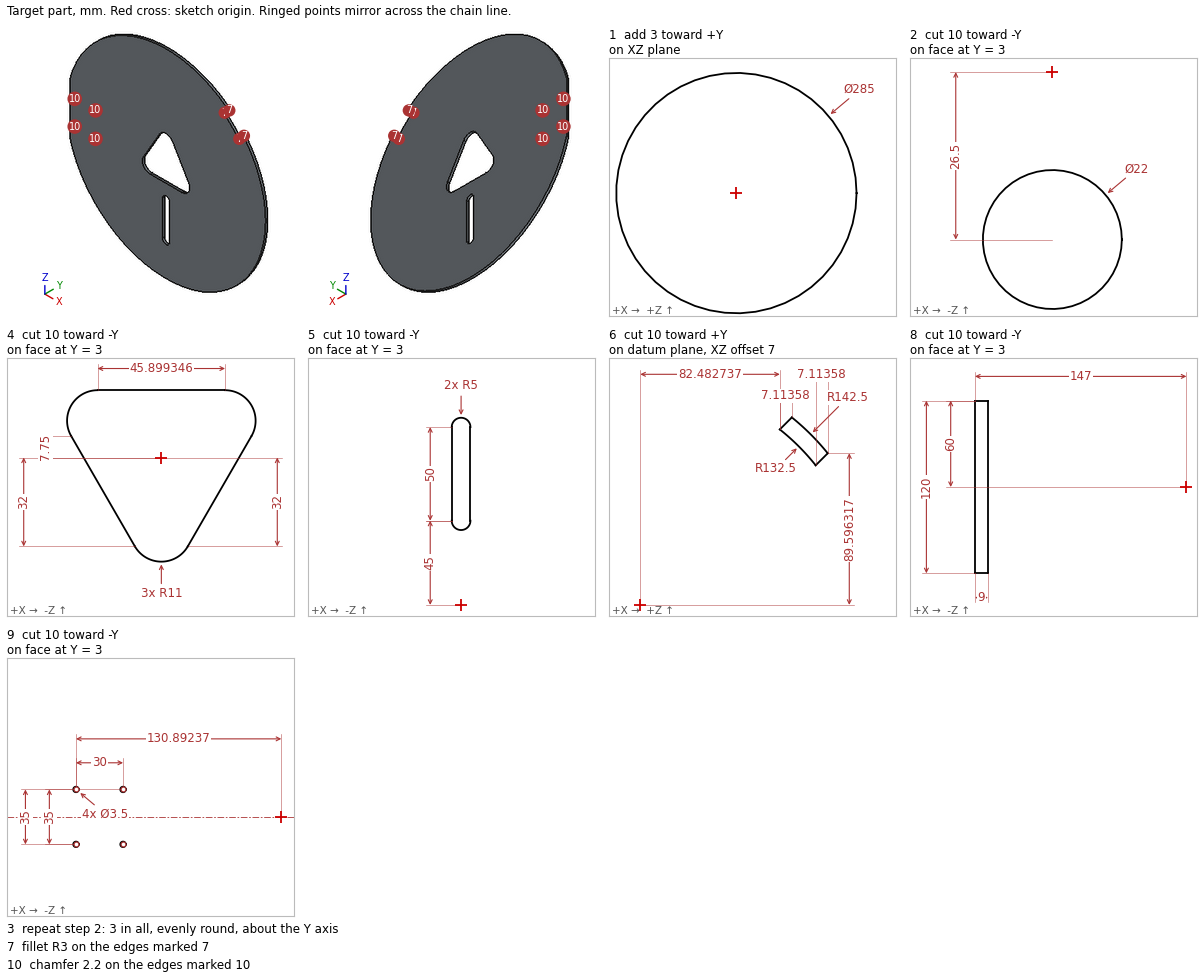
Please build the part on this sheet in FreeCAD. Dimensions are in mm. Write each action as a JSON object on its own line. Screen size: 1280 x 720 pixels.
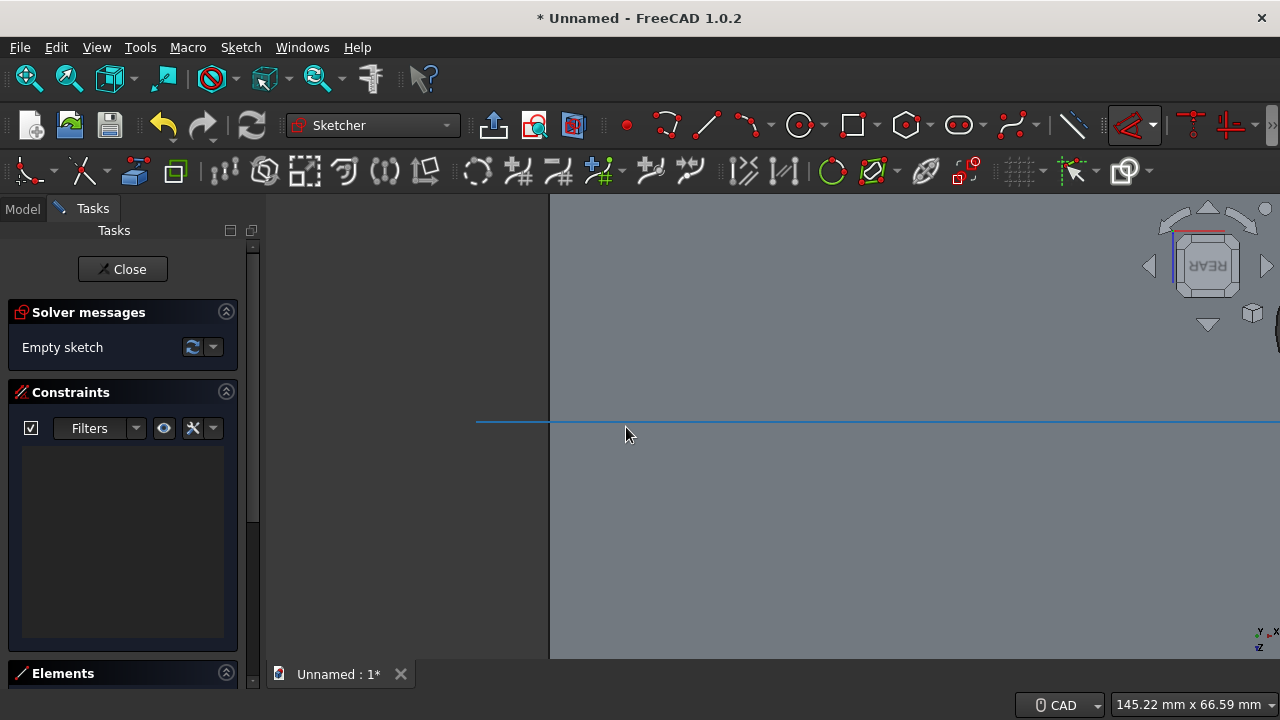
{"action": "left_click", "coordinate": [800, 126]}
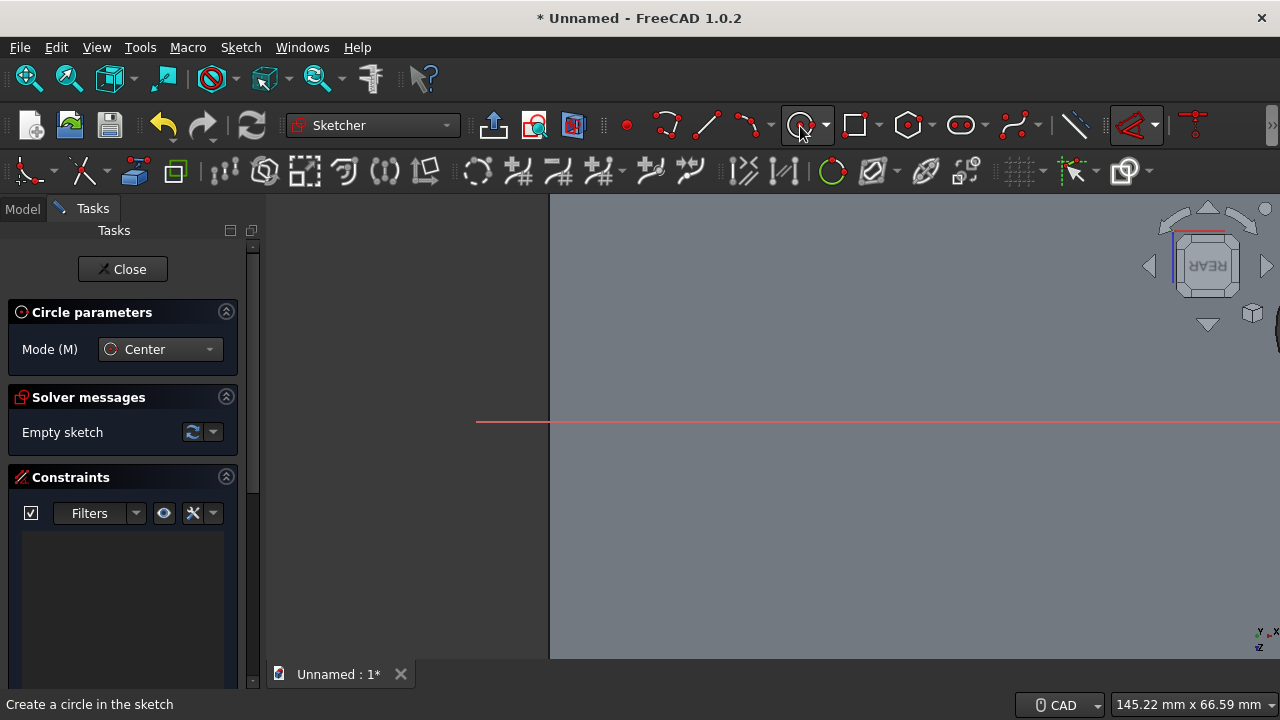
{"action": "scroll", "coordinate": [599, 299], "scroll_direction": "up", "scroll_amount": 4}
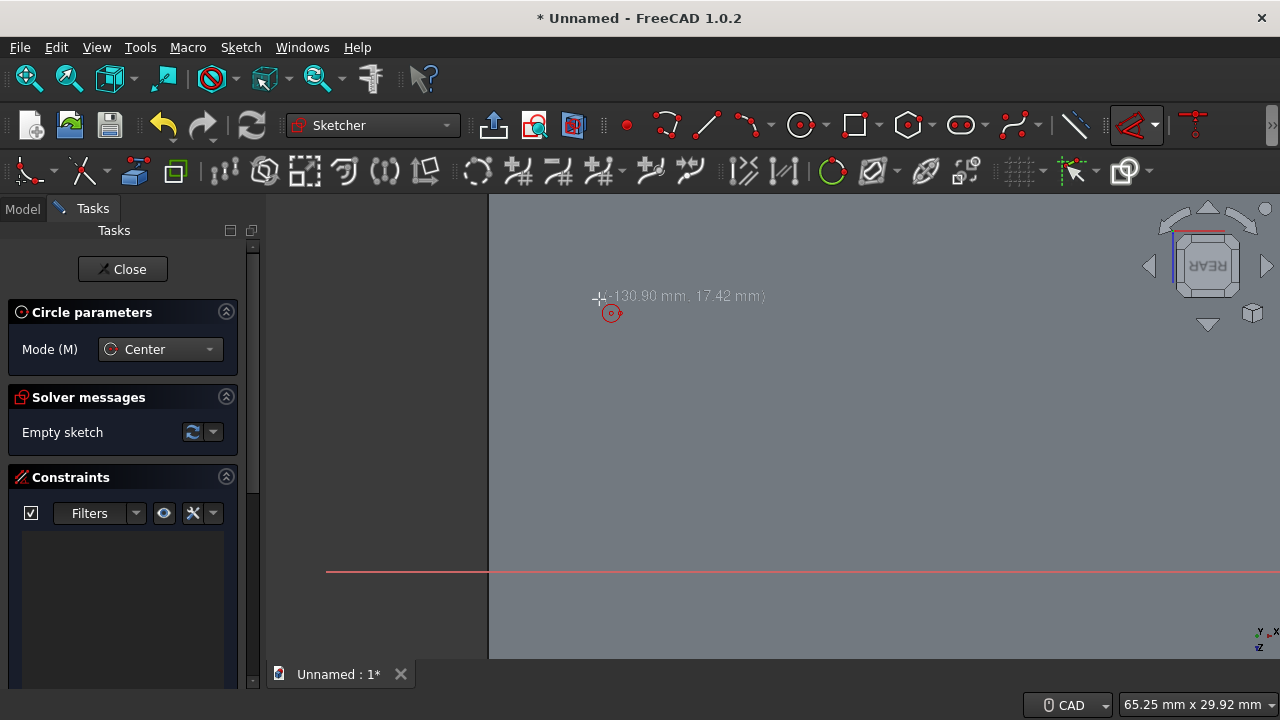
{"action": "left_click", "coordinate": [599, 300]}
{"action": "left_click", "coordinate": [618, 281]}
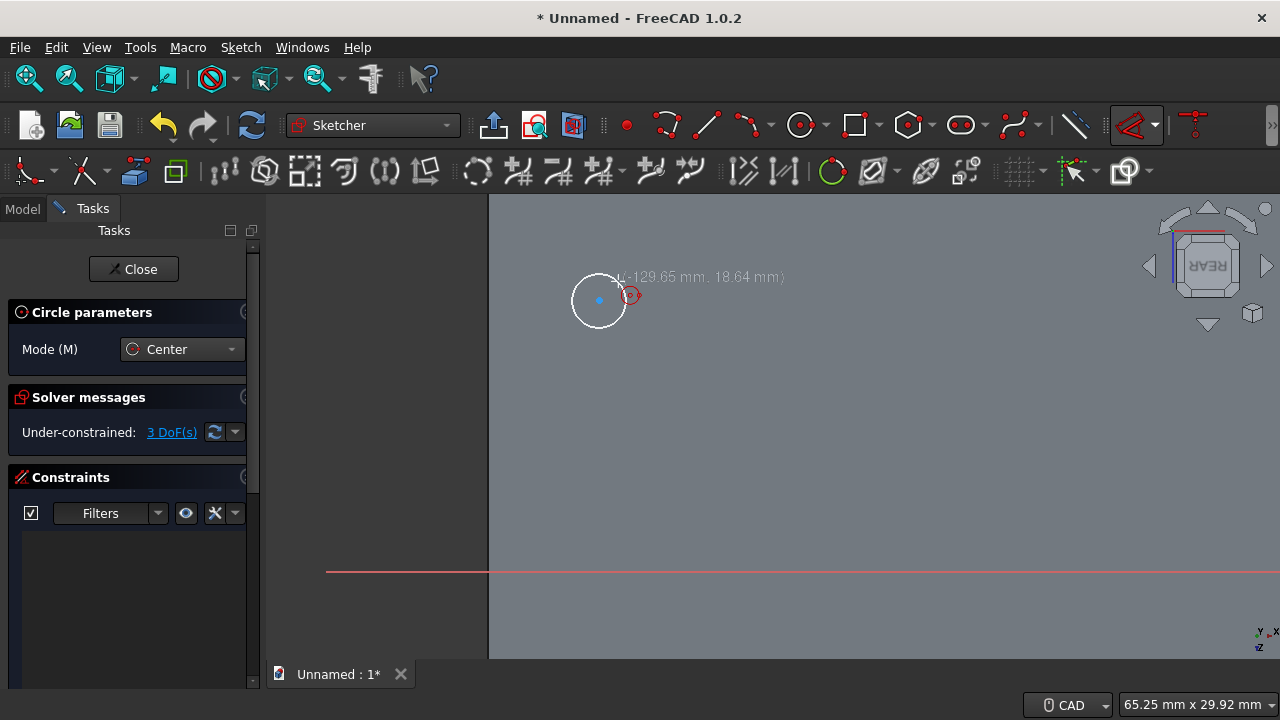
{"action": "left_click", "coordinate": [1065, 300]}
{"action": "left_click", "coordinate": [1084, 281]}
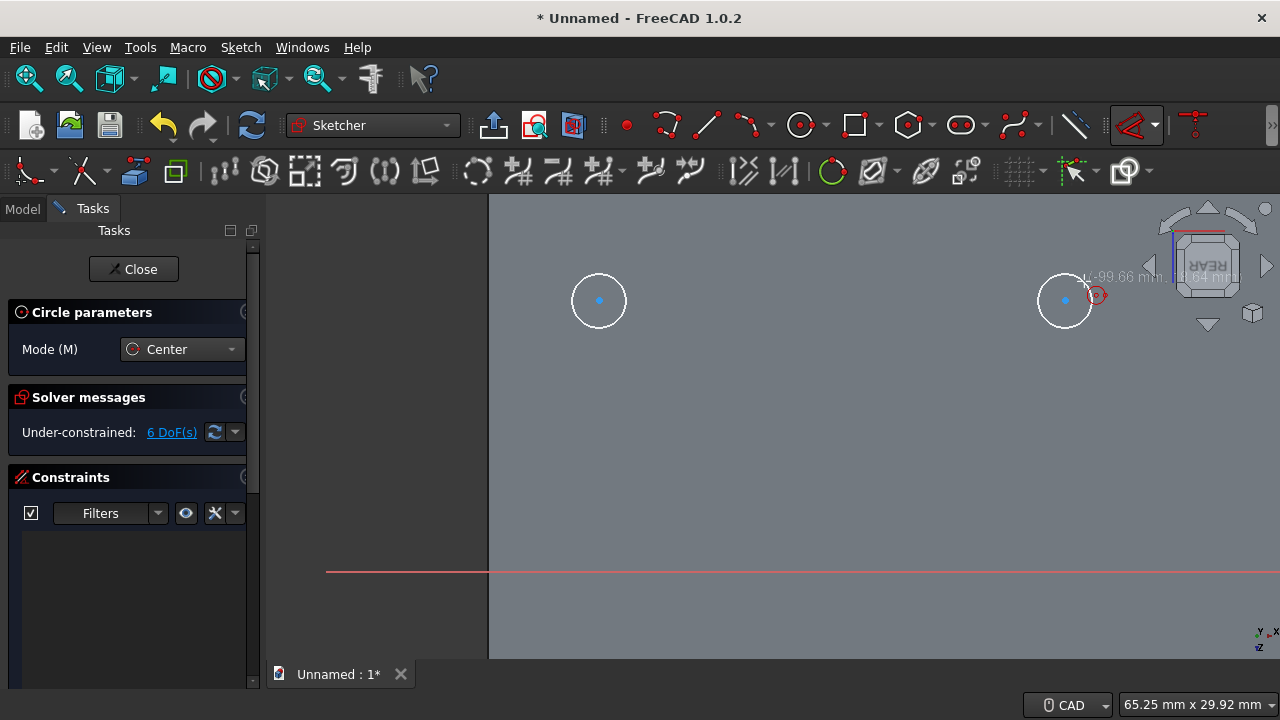
{"action": "scroll", "coordinate": [601, 308], "scroll_direction": "down", "scroll_amount": 4}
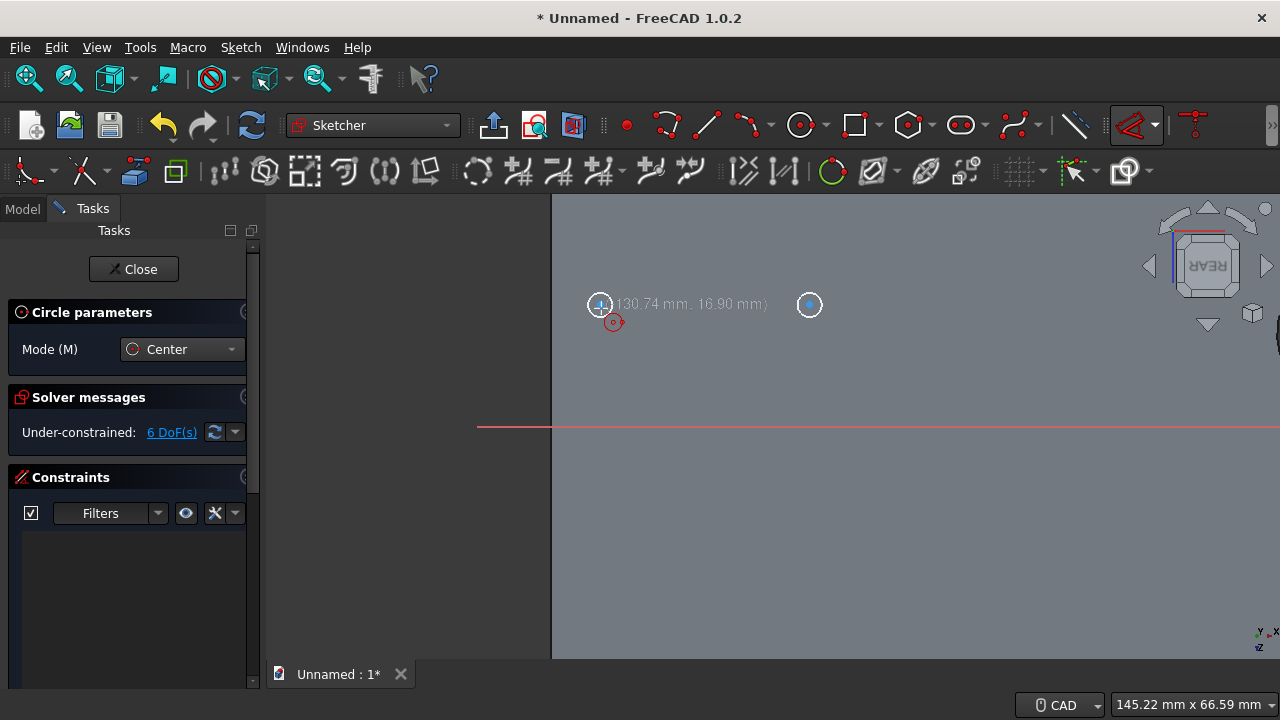
{"action": "scroll", "coordinate": [600, 549], "scroll_direction": "up", "scroll_amount": 4}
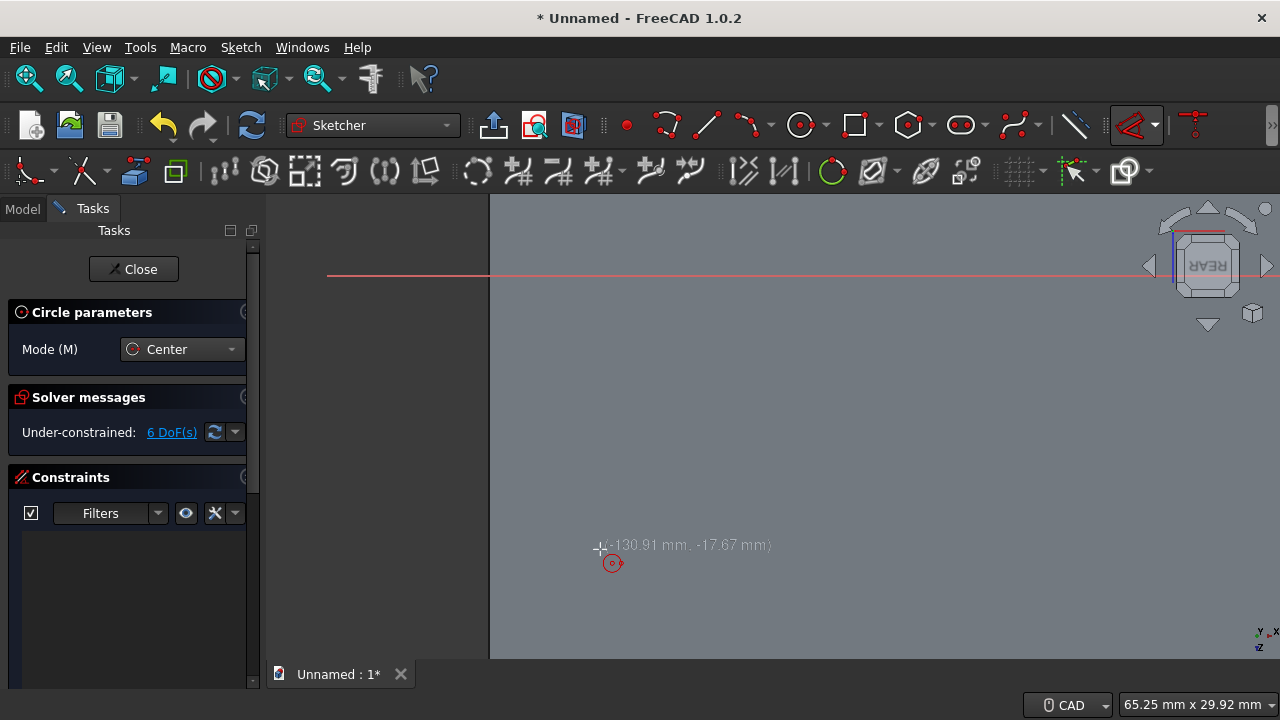
{"action": "left_click", "coordinate": [600, 548]}
{"action": "left_click", "coordinate": [619, 528]}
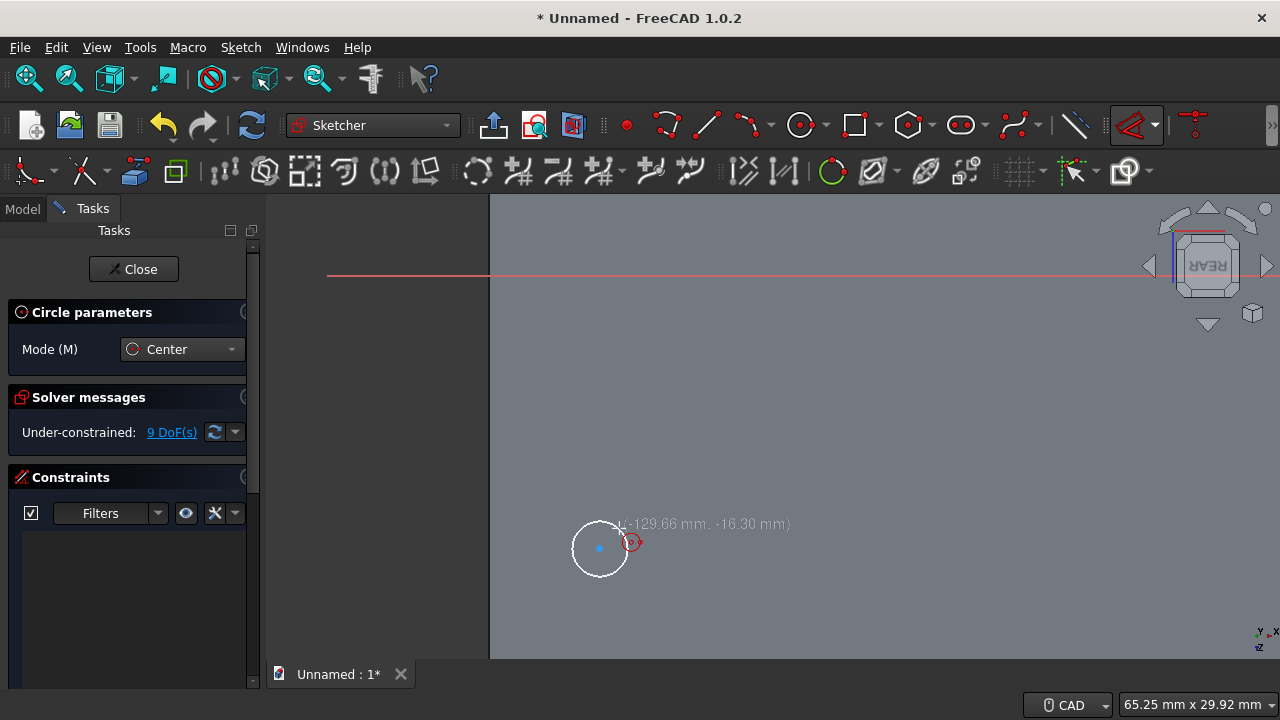
{"action": "left_click", "coordinate": [1066, 548]}
{"action": "left_click", "coordinate": [1085, 528]}
{"action": "key", "text": "Escape"}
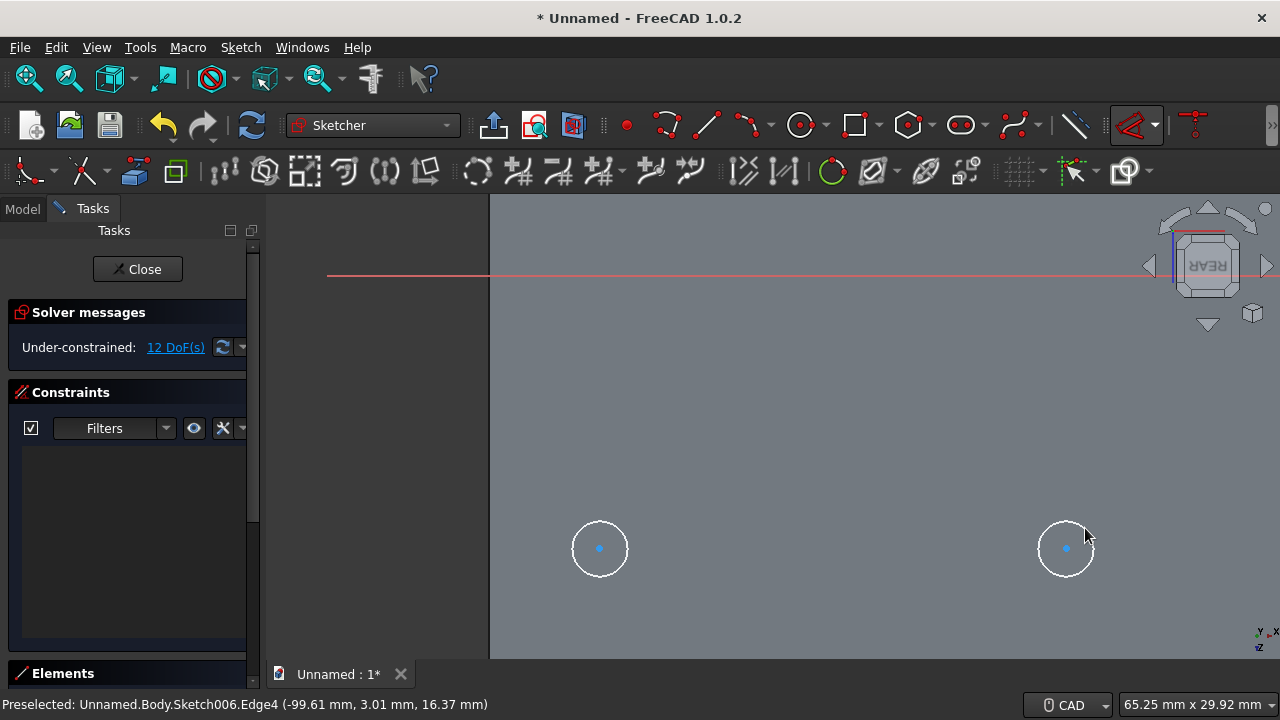
{"action": "scroll", "coordinate": [600, 550], "scroll_direction": "down", "scroll_amount": 4}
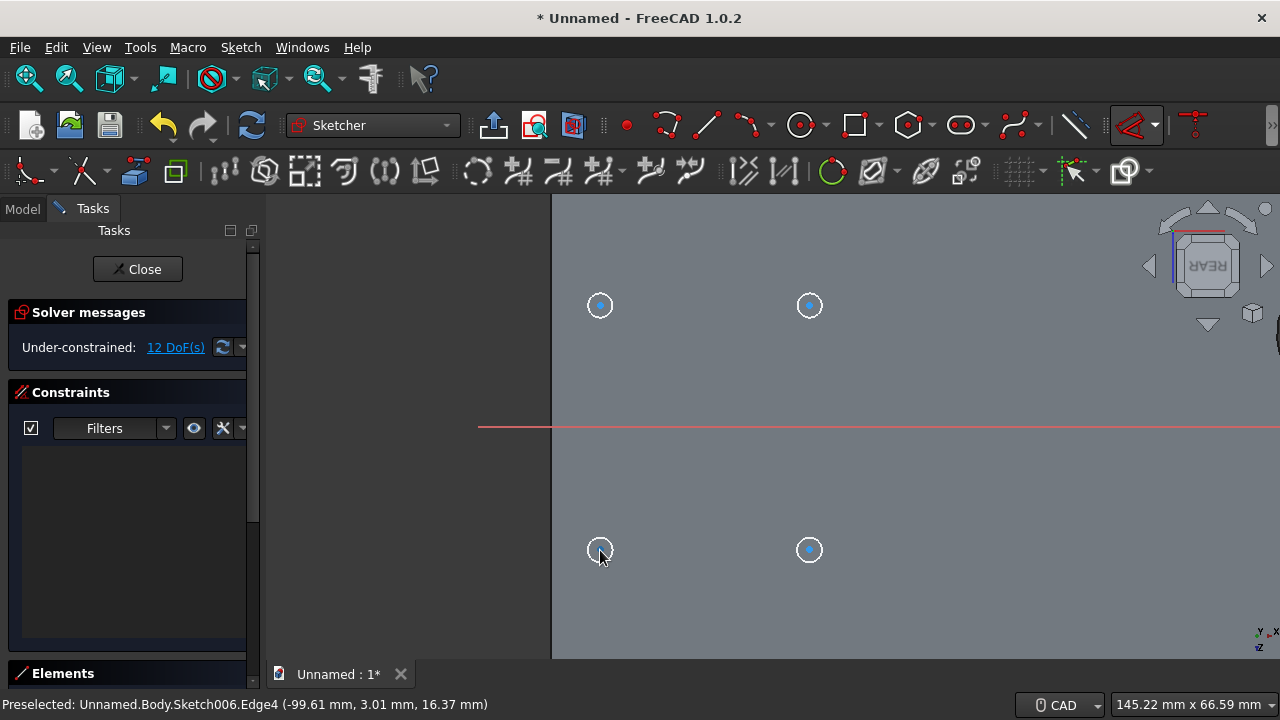
{"action": "left_click", "coordinate": [609, 297]}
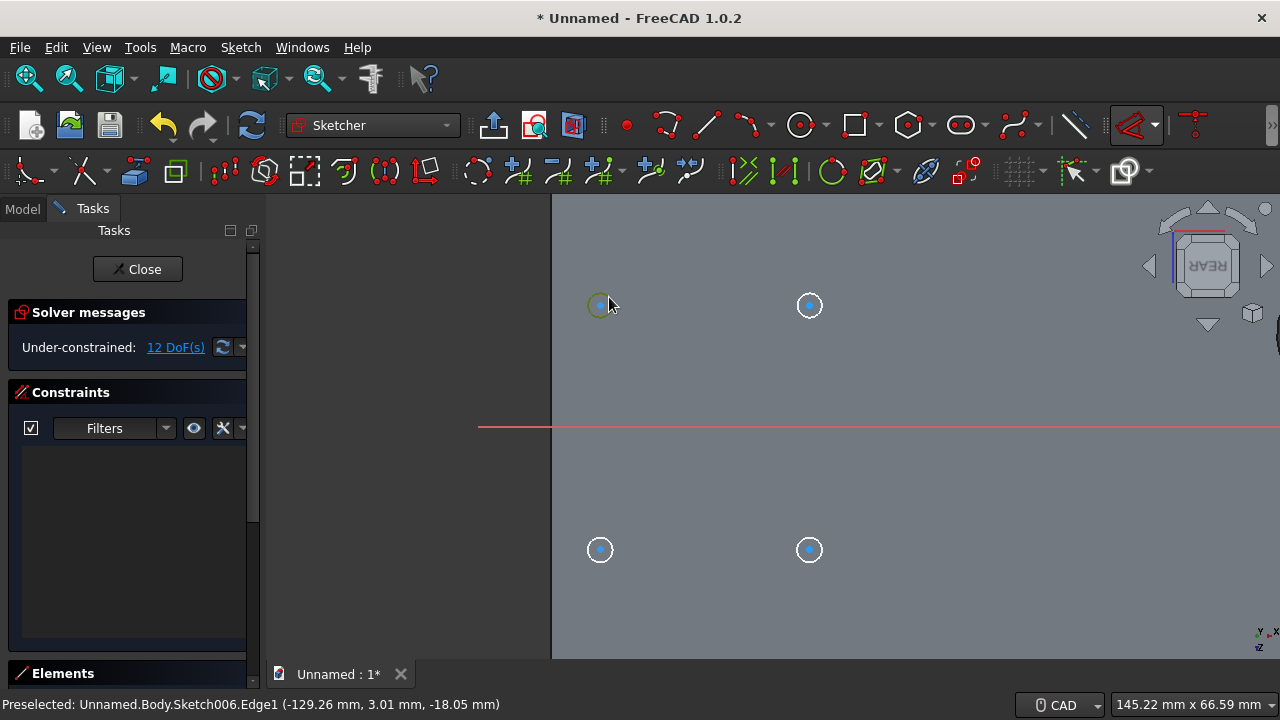
{"action": "left_click", "coordinate": [818, 297]}